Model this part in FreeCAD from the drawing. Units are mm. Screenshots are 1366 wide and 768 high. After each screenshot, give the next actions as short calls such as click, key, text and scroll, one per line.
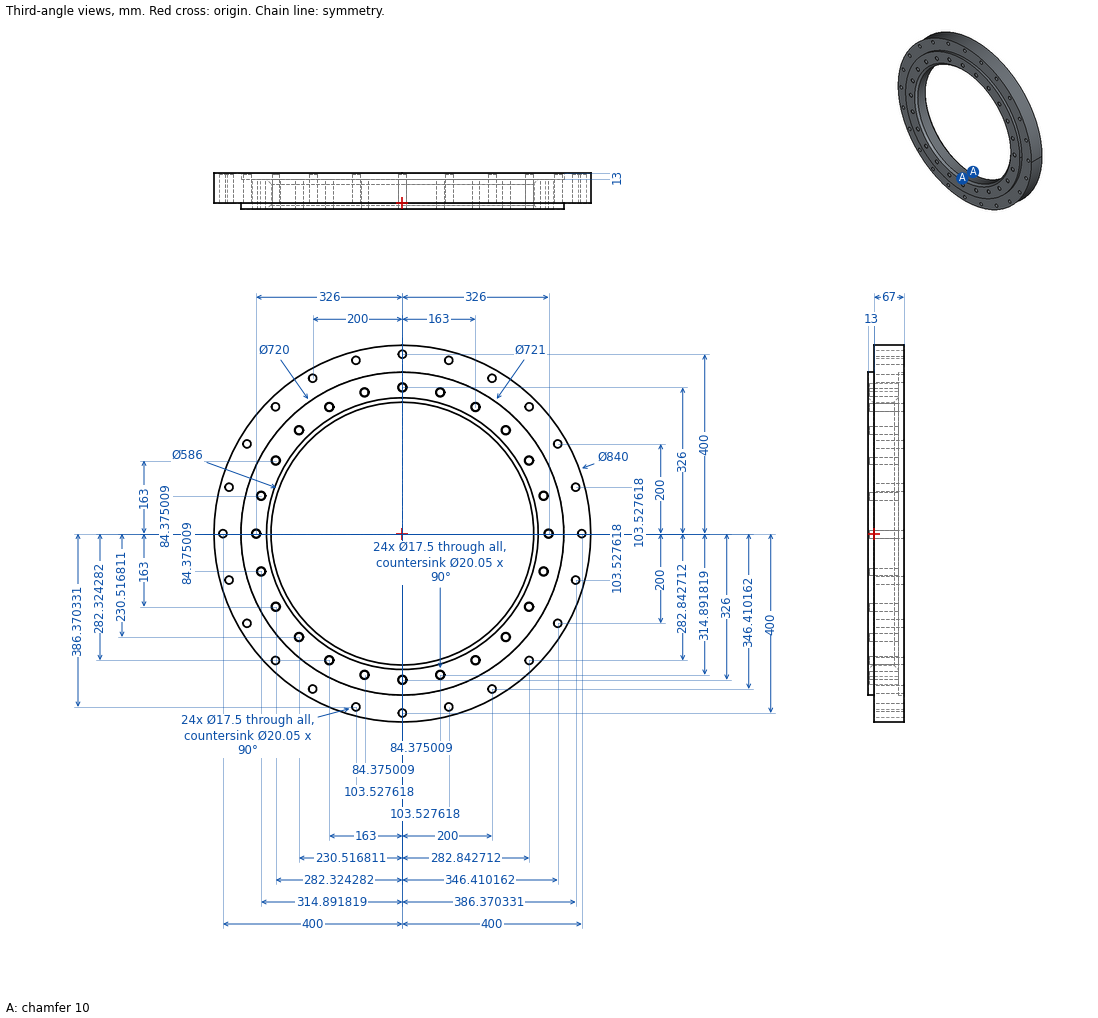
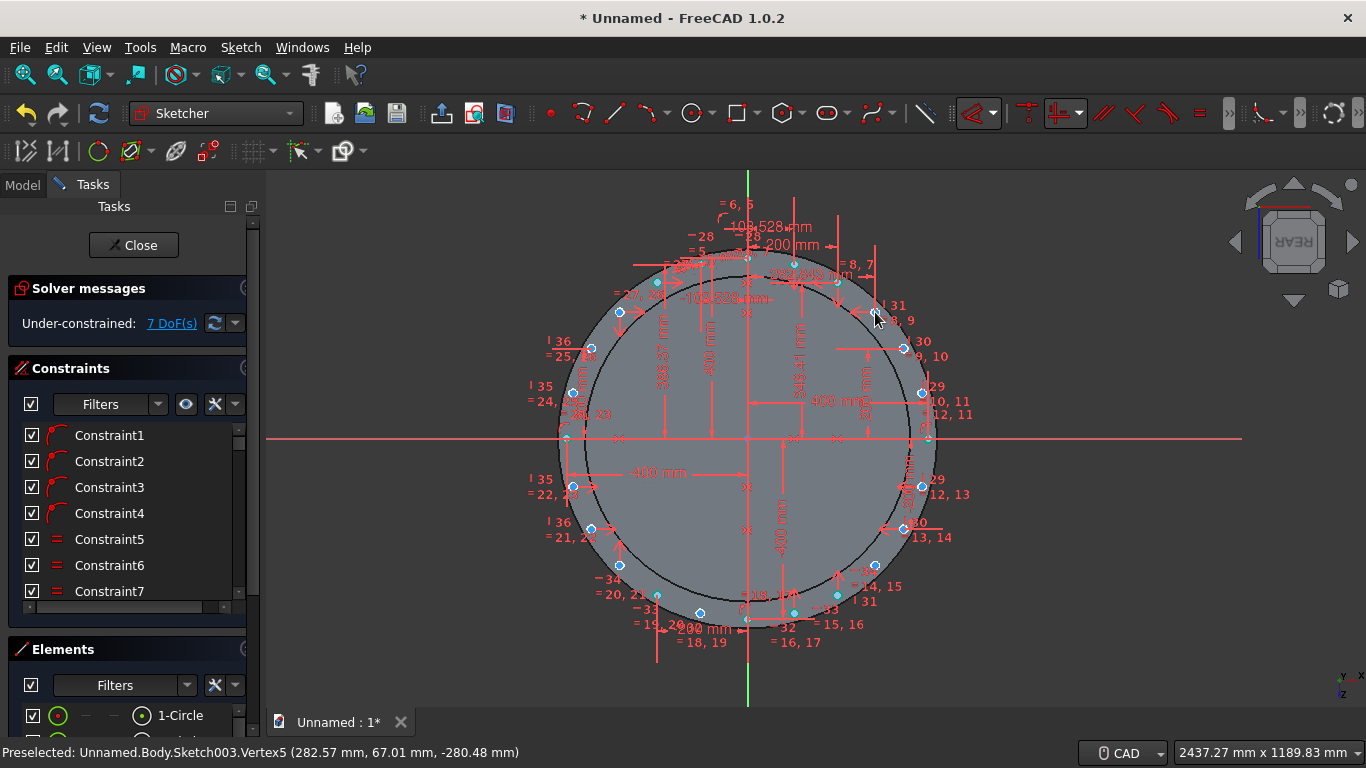
click(875, 312)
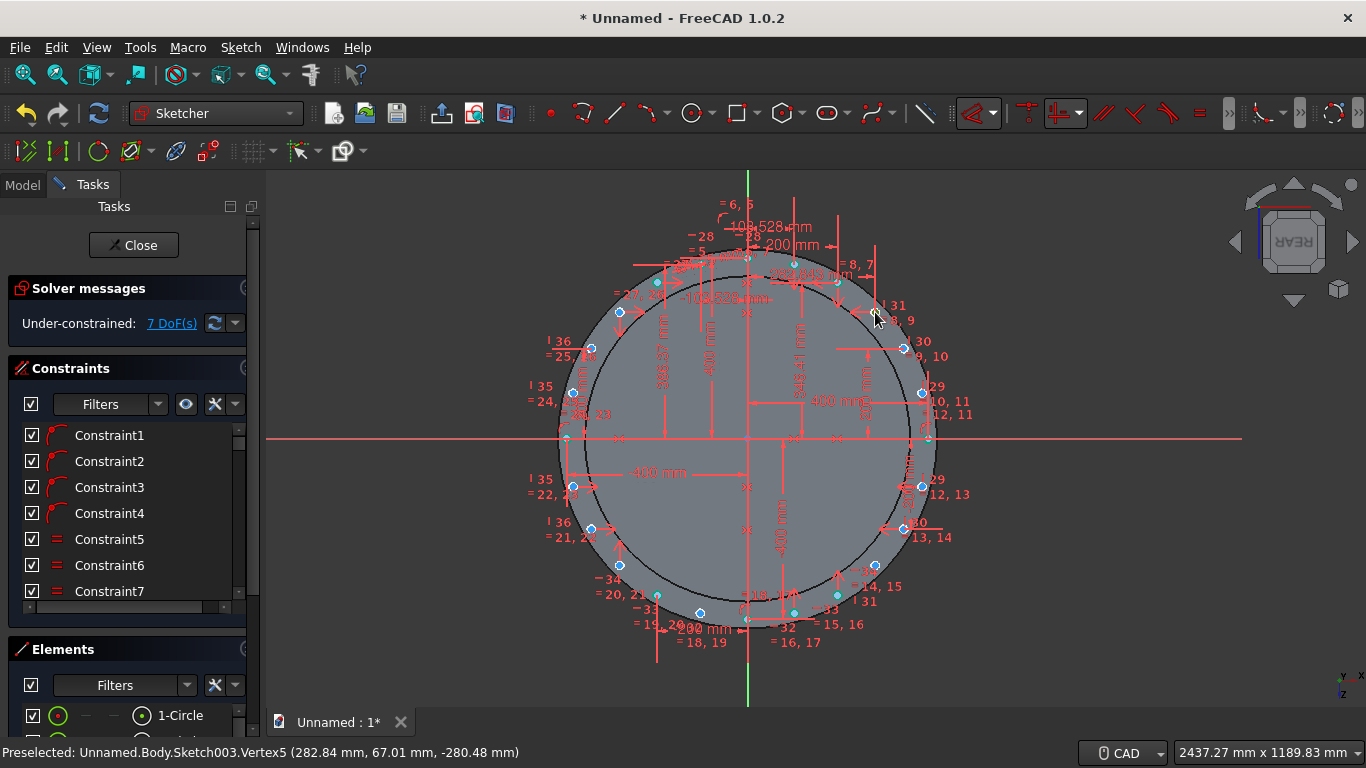
key(i)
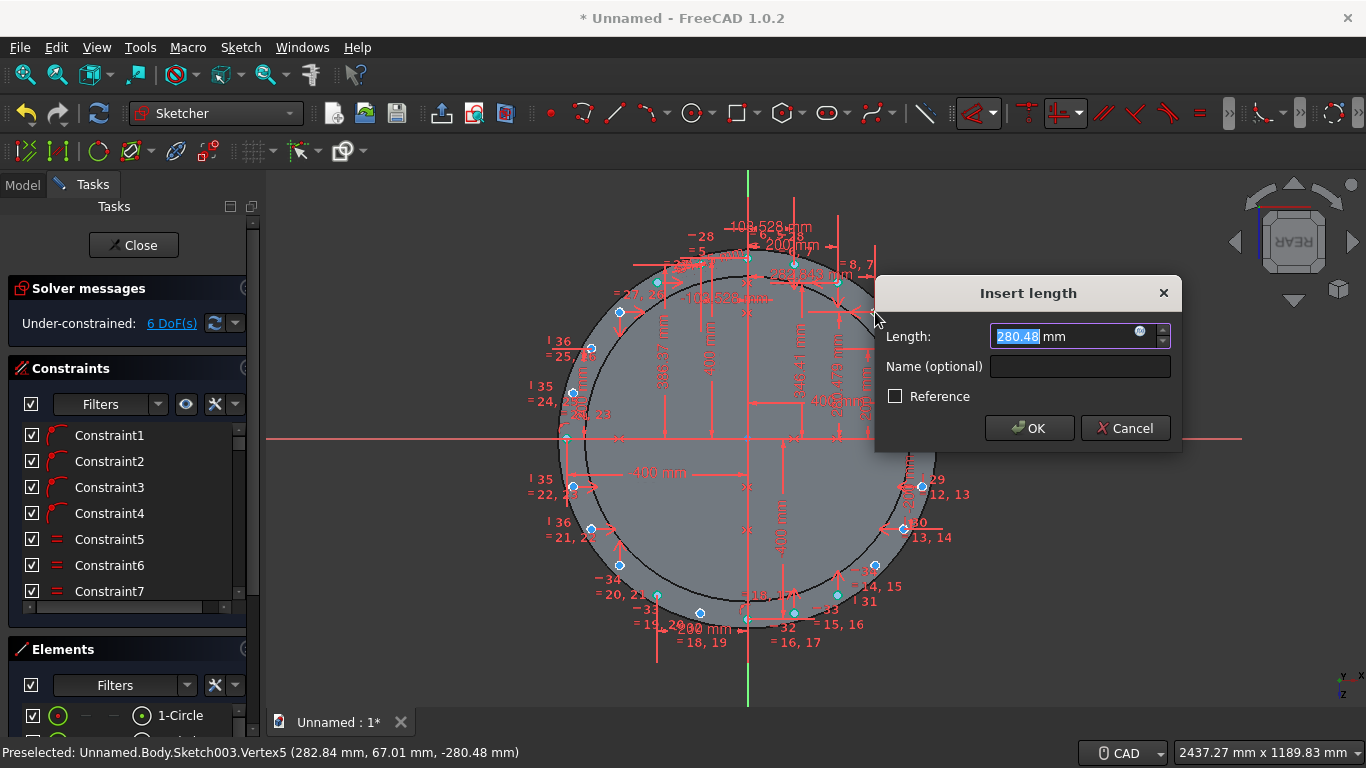
text(282.842712)
key(Return)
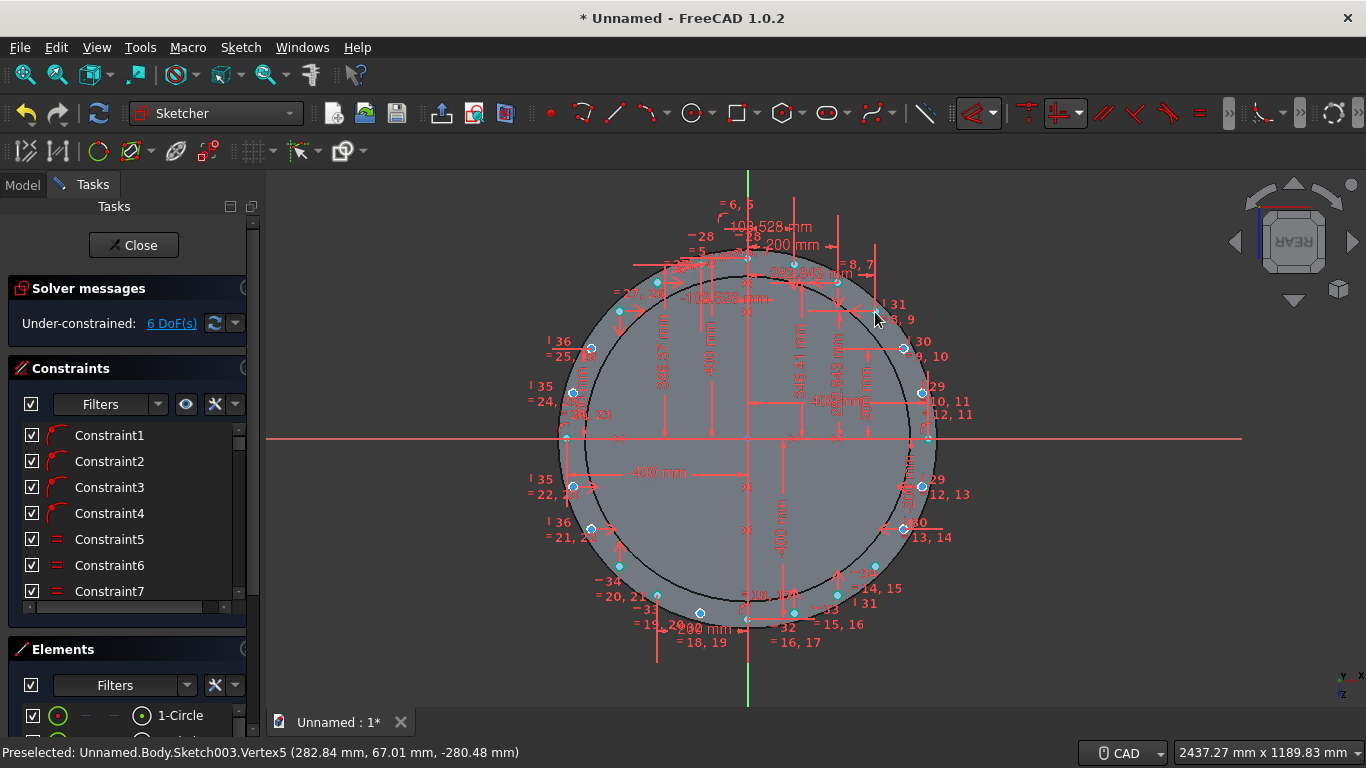
click(904, 349)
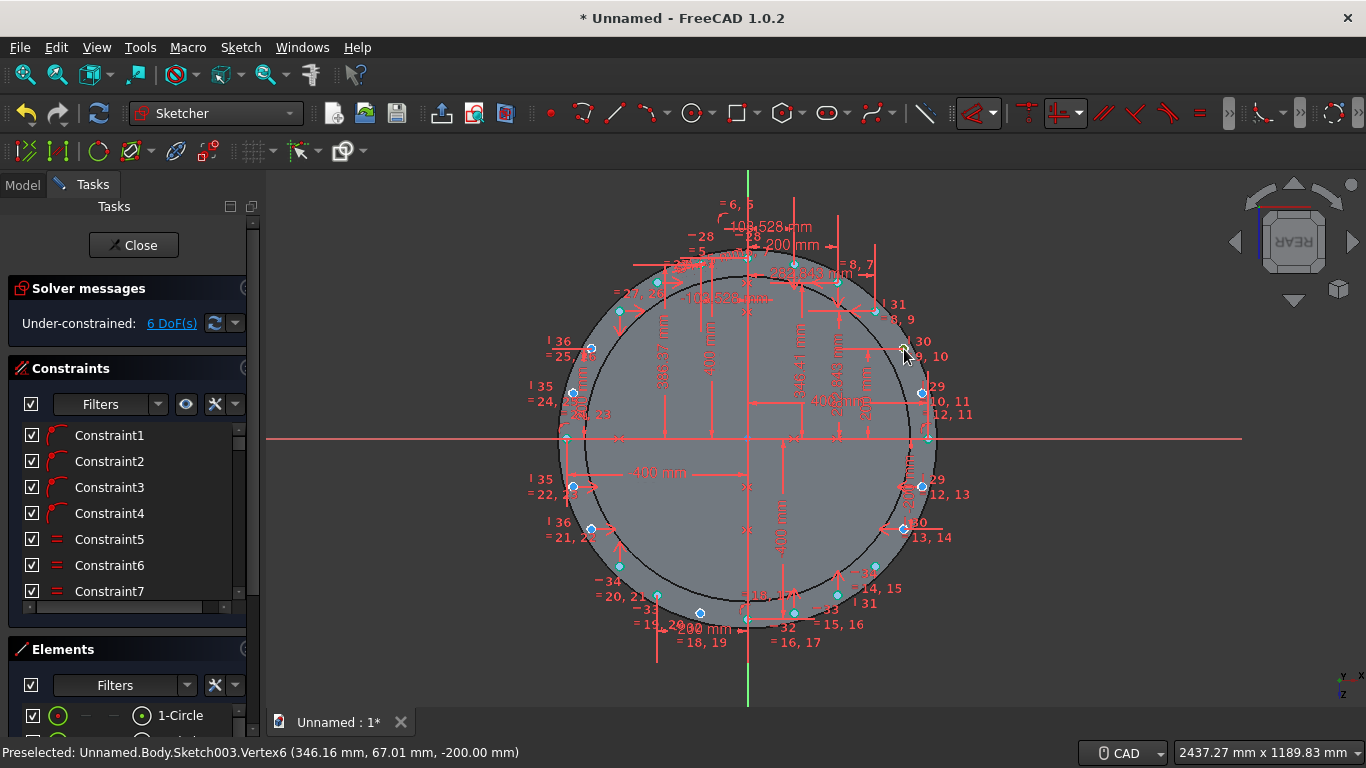
key(l)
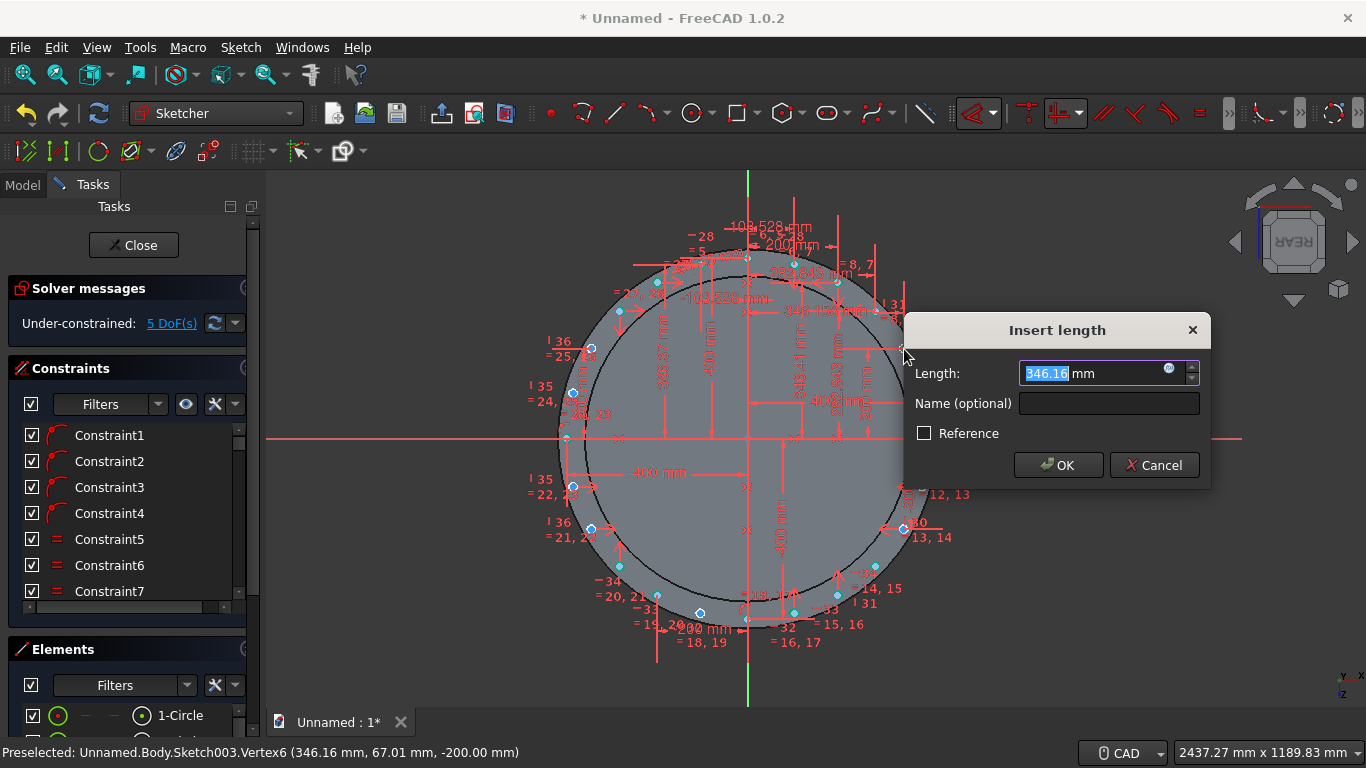
text(346.410162)
key(Return)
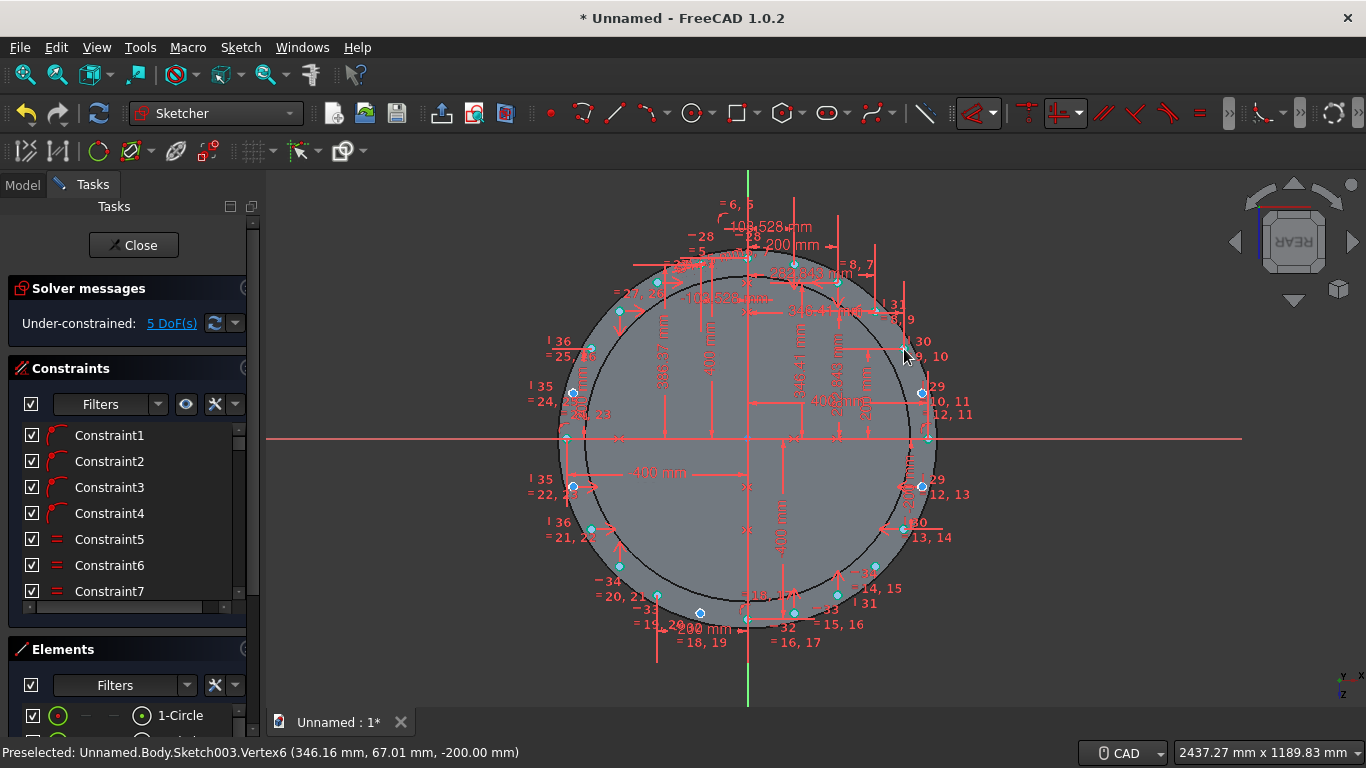
click(922, 393)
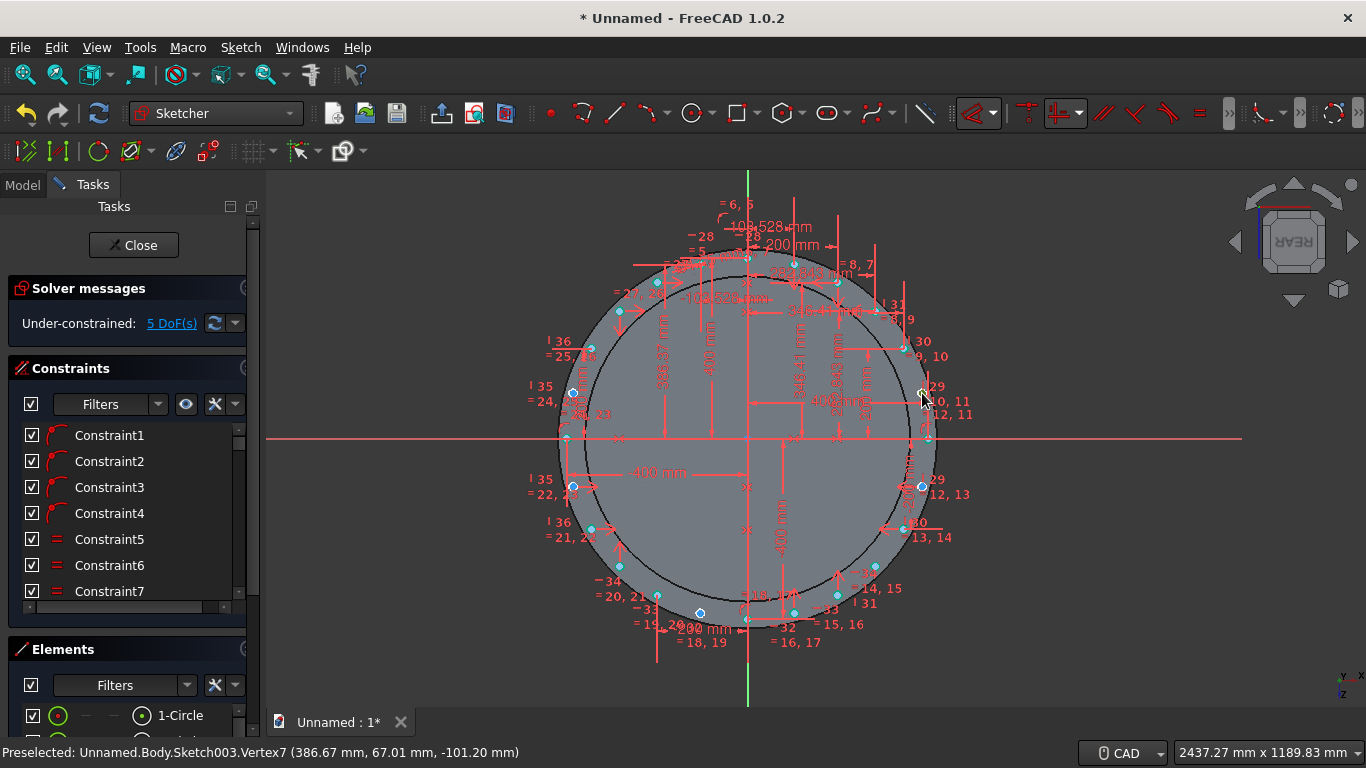
key(l)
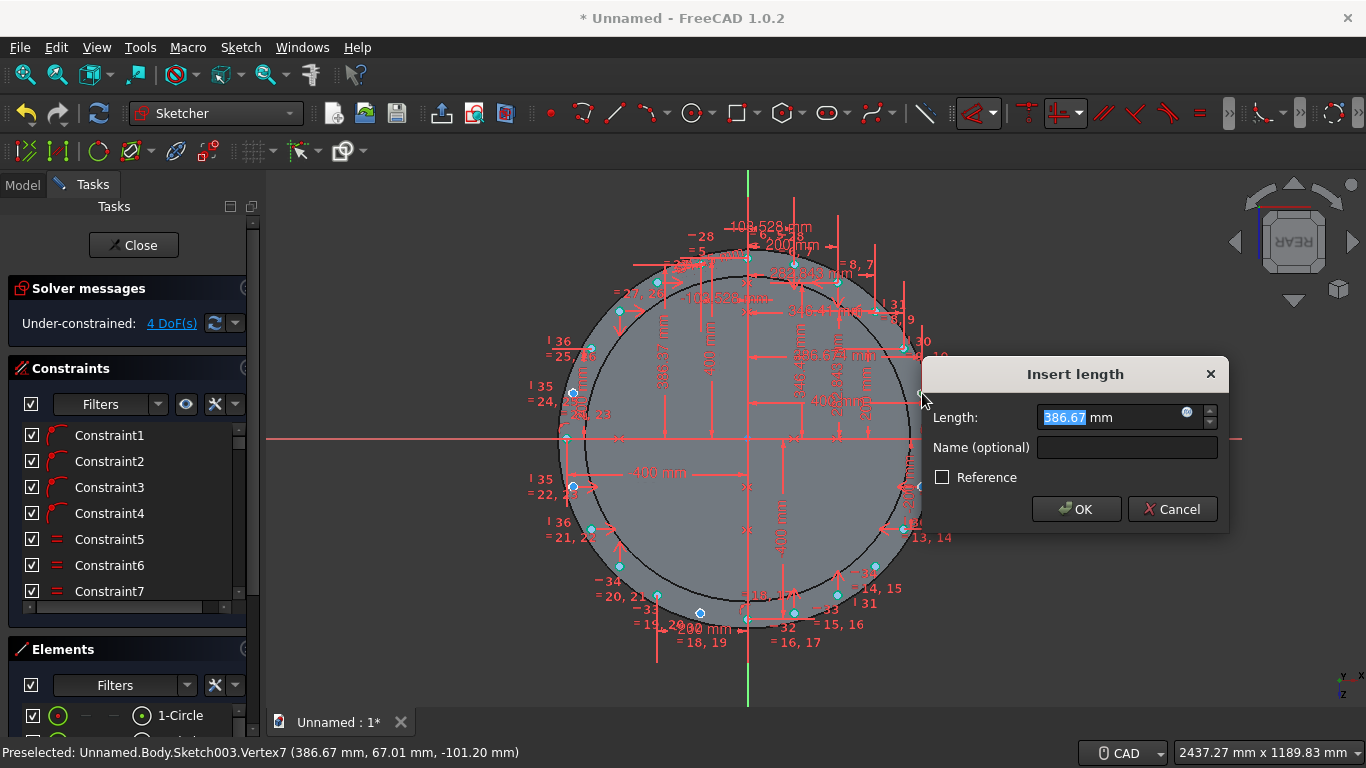
text(386.370331)
key(Return)